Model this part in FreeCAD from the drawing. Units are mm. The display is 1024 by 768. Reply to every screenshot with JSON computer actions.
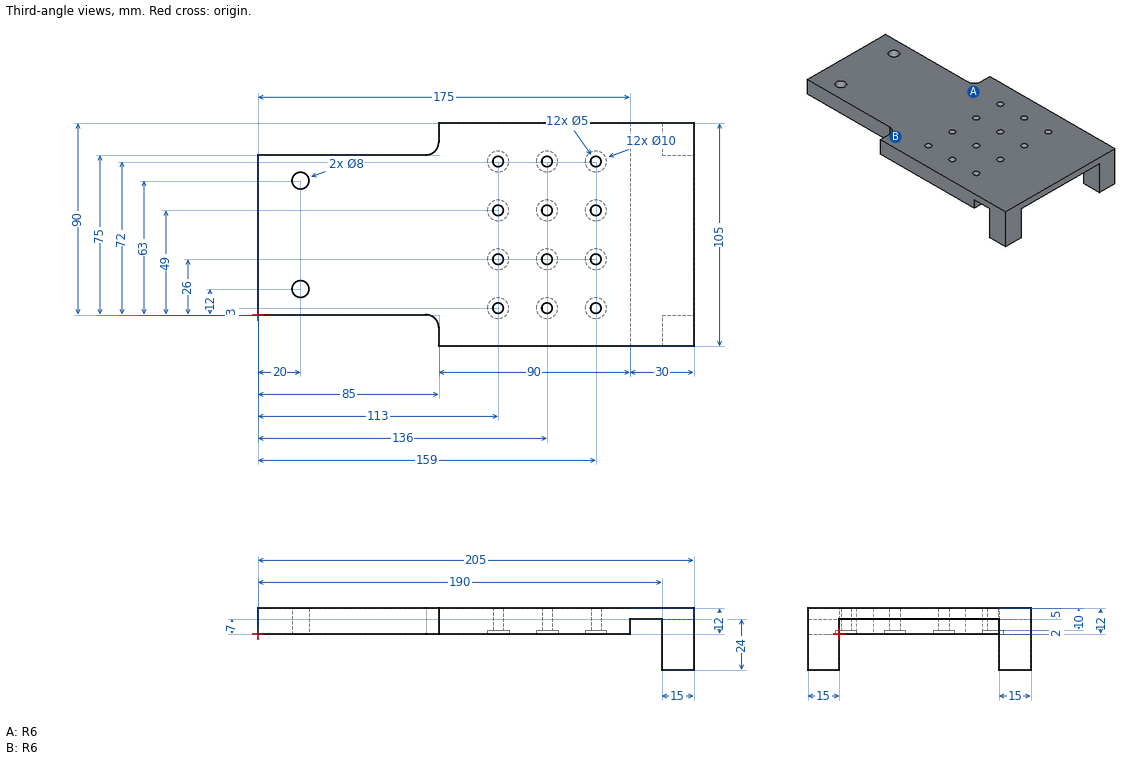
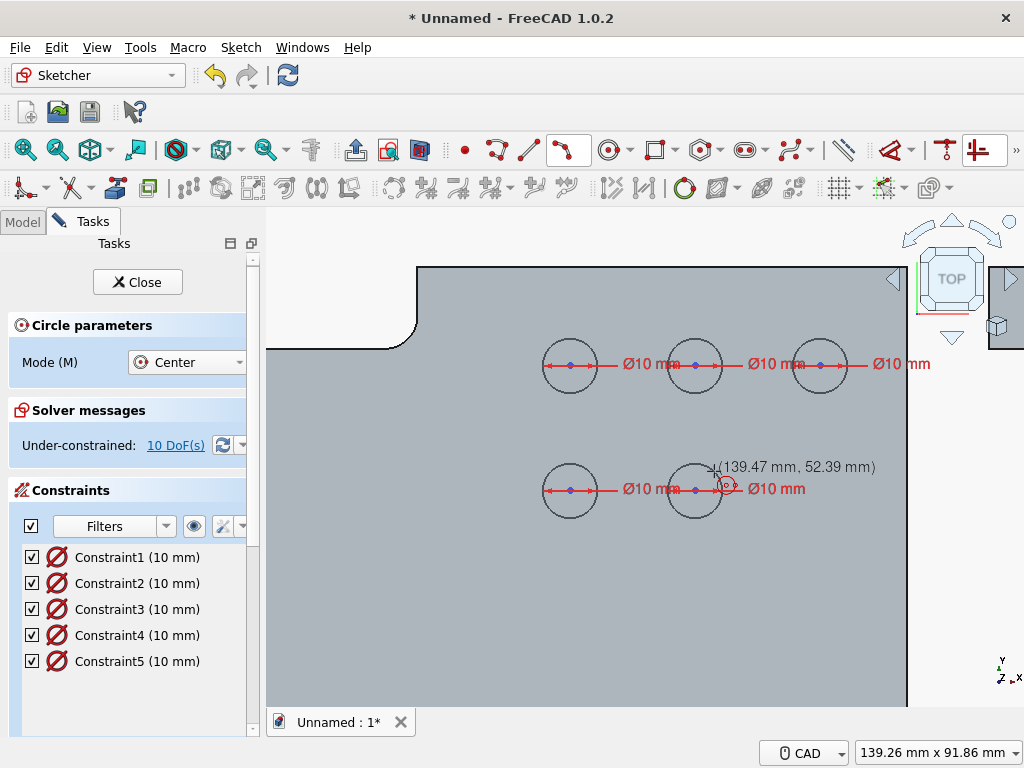
{"action": "left_click", "coordinate": [820, 490]}
{"action": "mouse_move", "coordinate": [840, 471]}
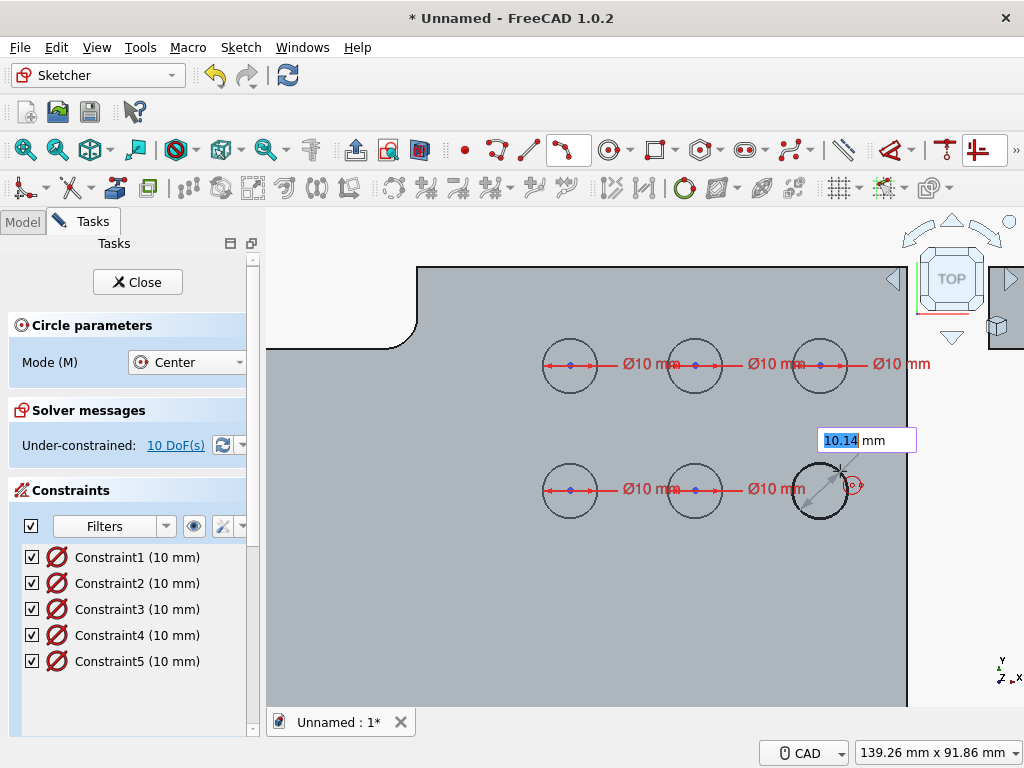
{"action": "type", "text": "10"}
{"action": "key", "text": "Return"}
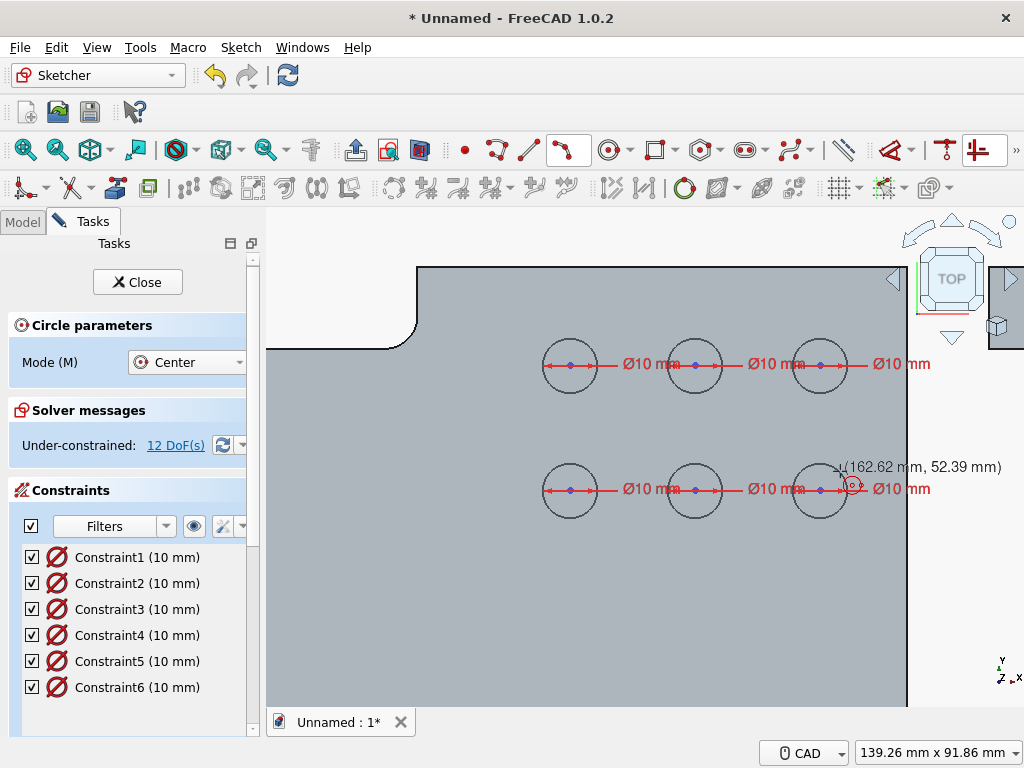
{"action": "left_click", "coordinate": [820, 616]}
{"action": "mouse_move", "coordinate": [840, 596]}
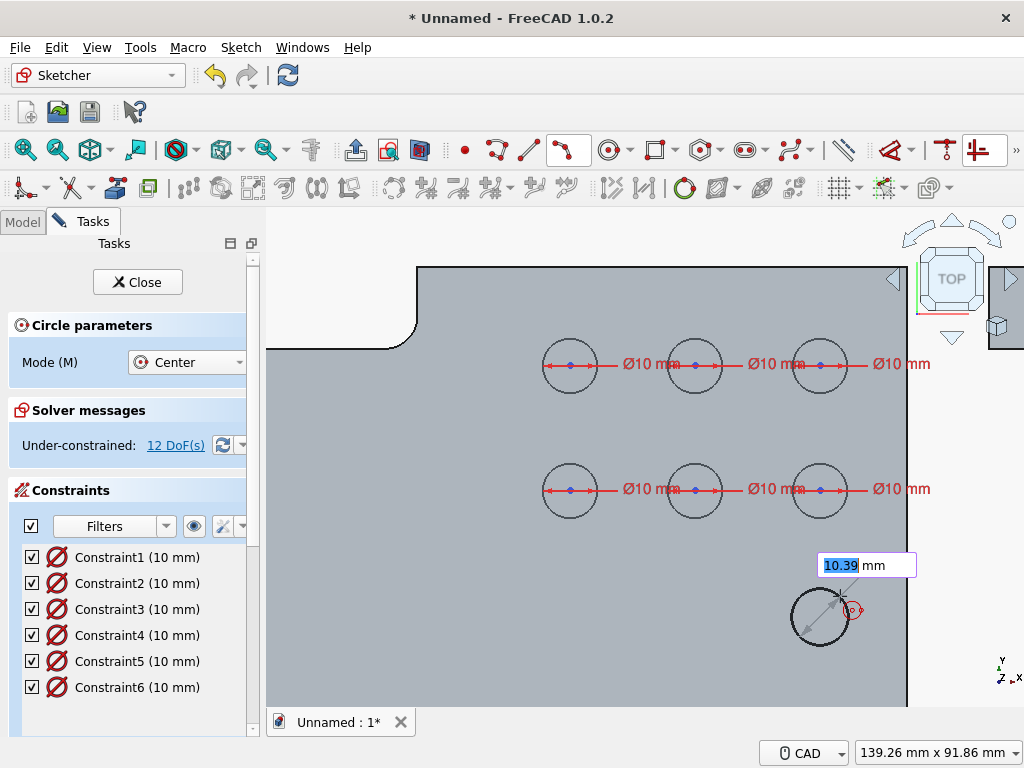
{"action": "type", "text": "10"}
{"action": "key", "text": "Return"}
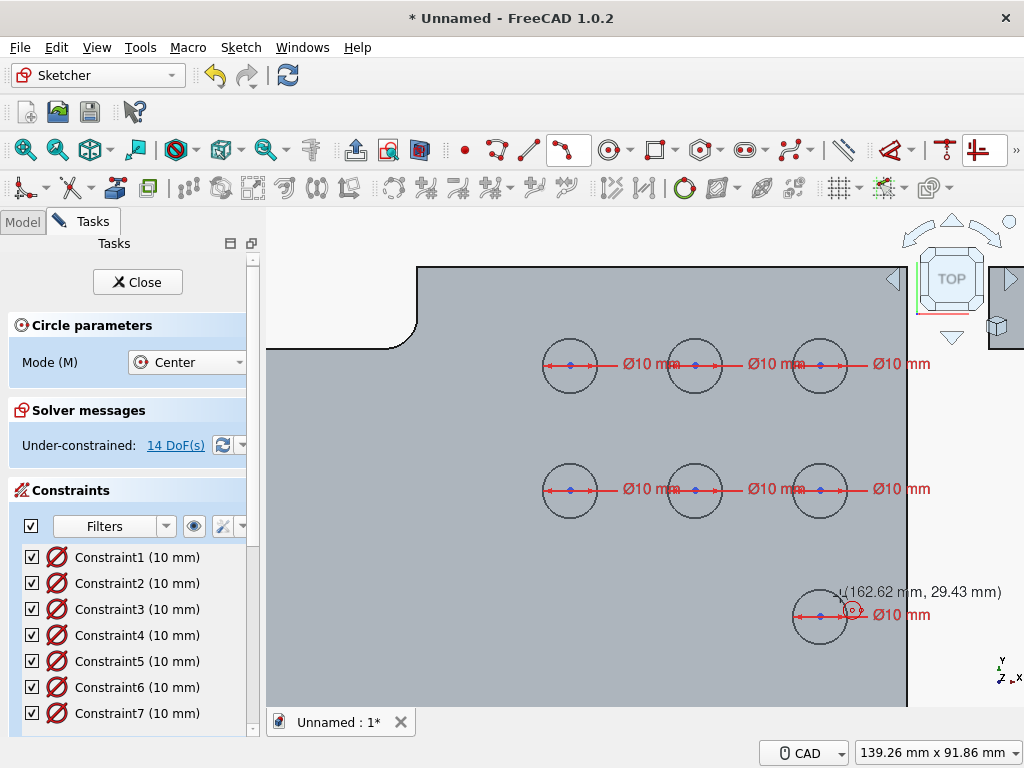
{"action": "left_click", "coordinate": [695, 616]}
{"action": "mouse_move", "coordinate": [714, 596]}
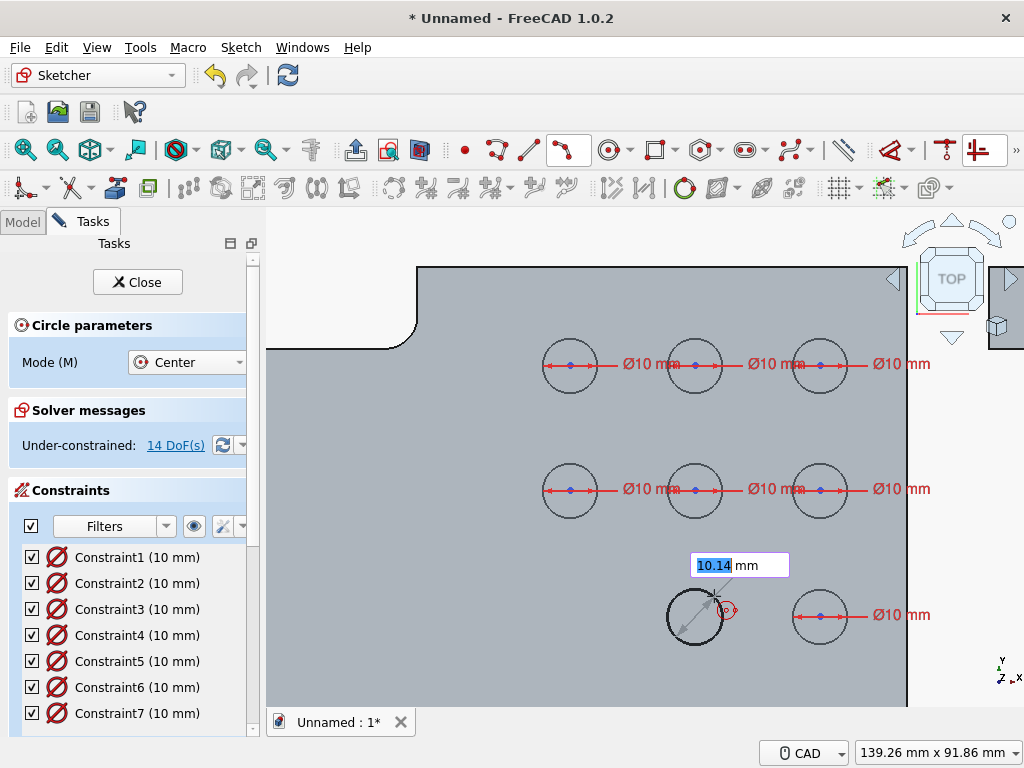
{"action": "type", "text": "10"}
{"action": "key", "text": "Return"}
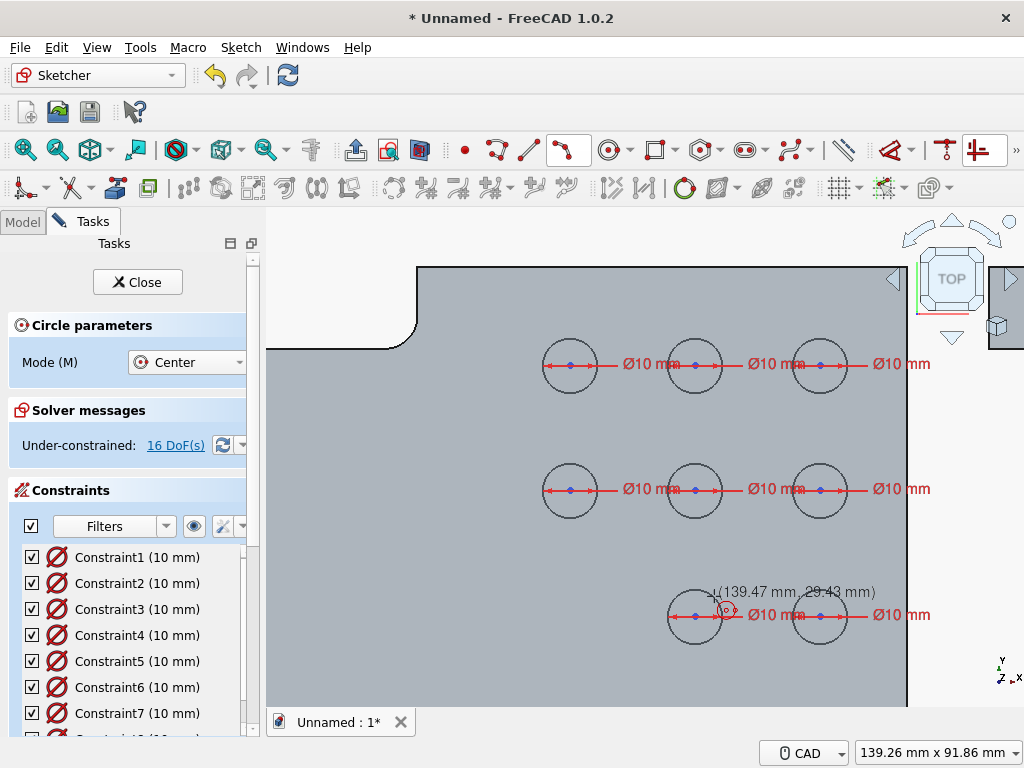
{"action": "left_click", "coordinate": [570, 616]}
{"action": "mouse_move", "coordinate": [589, 596]}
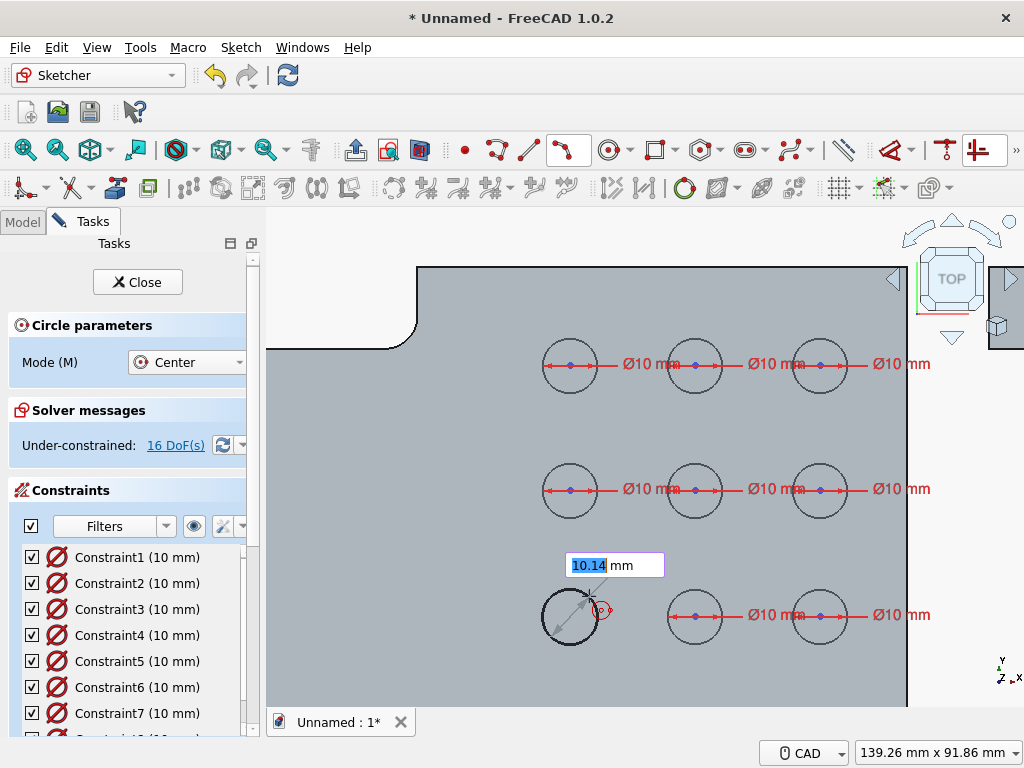
{"action": "type", "text": "10"}
{"action": "key", "text": "Return"}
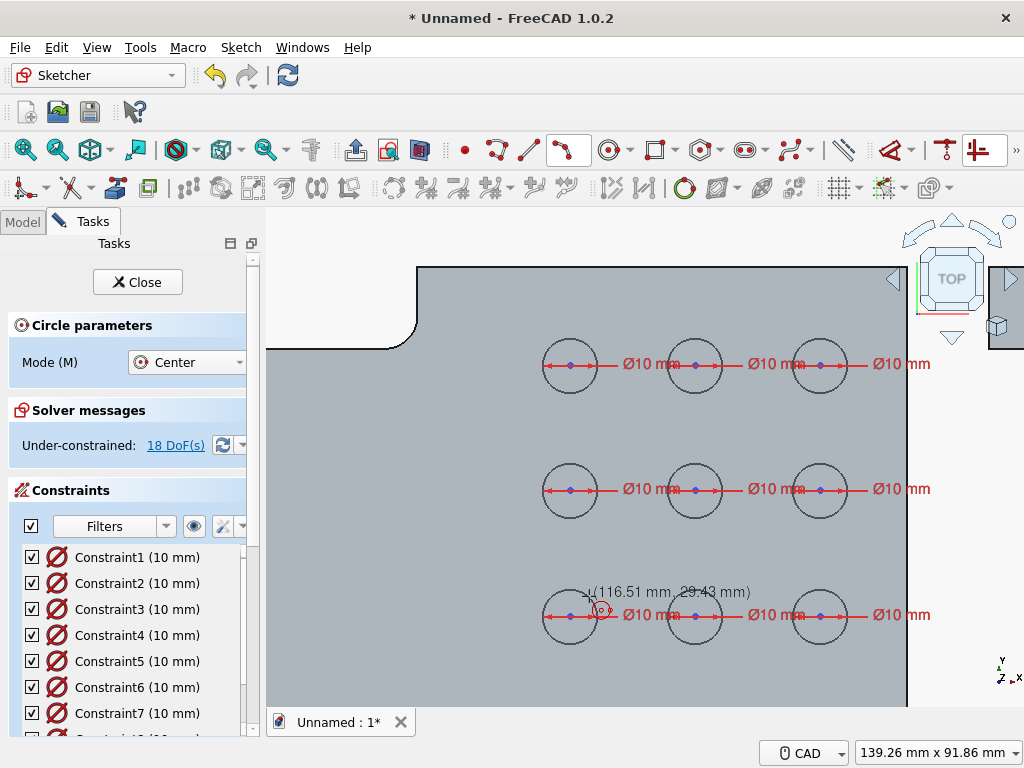
{"action": "scroll", "coordinate": [720, 379], "scroll_direction": "down", "scroll_amount": 4}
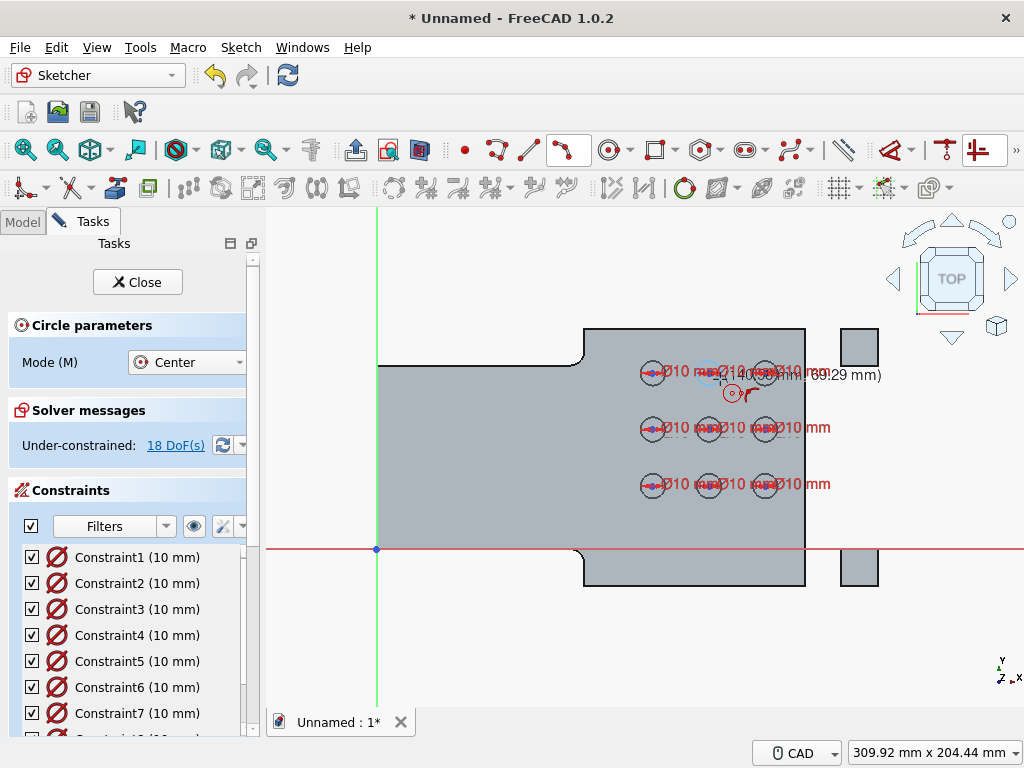
{"action": "scroll", "coordinate": [653, 542], "scroll_direction": "up", "scroll_amount": 4}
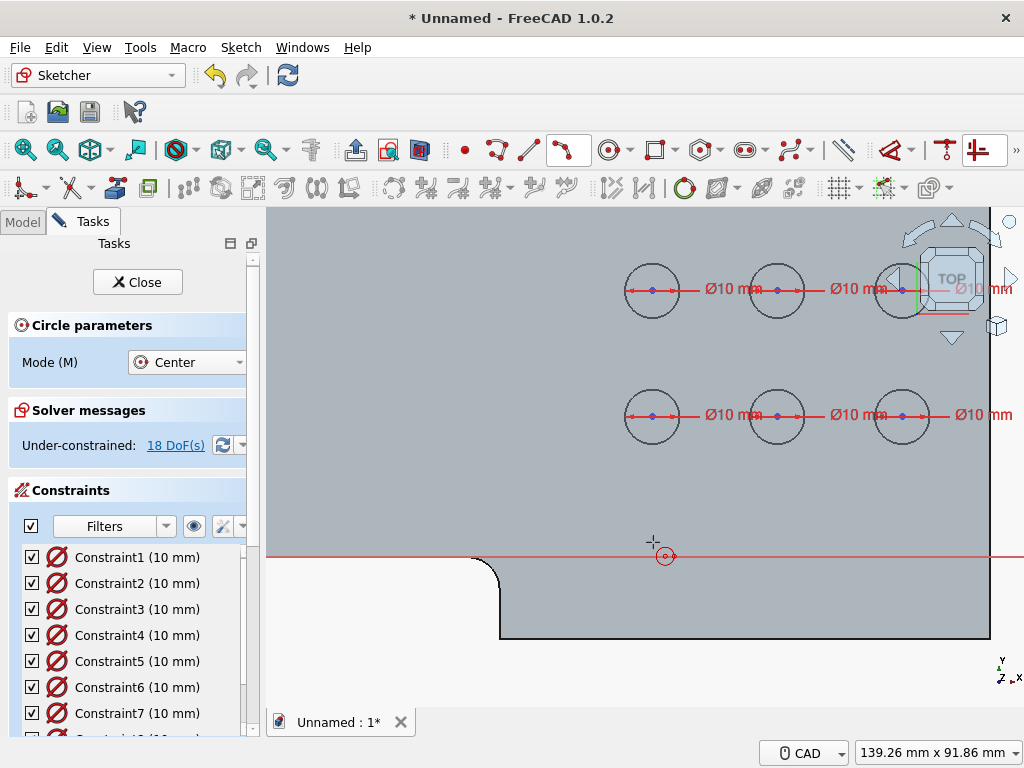
{"action": "left_click", "coordinate": [652, 541]}
{"action": "mouse_move", "coordinate": [671, 521]}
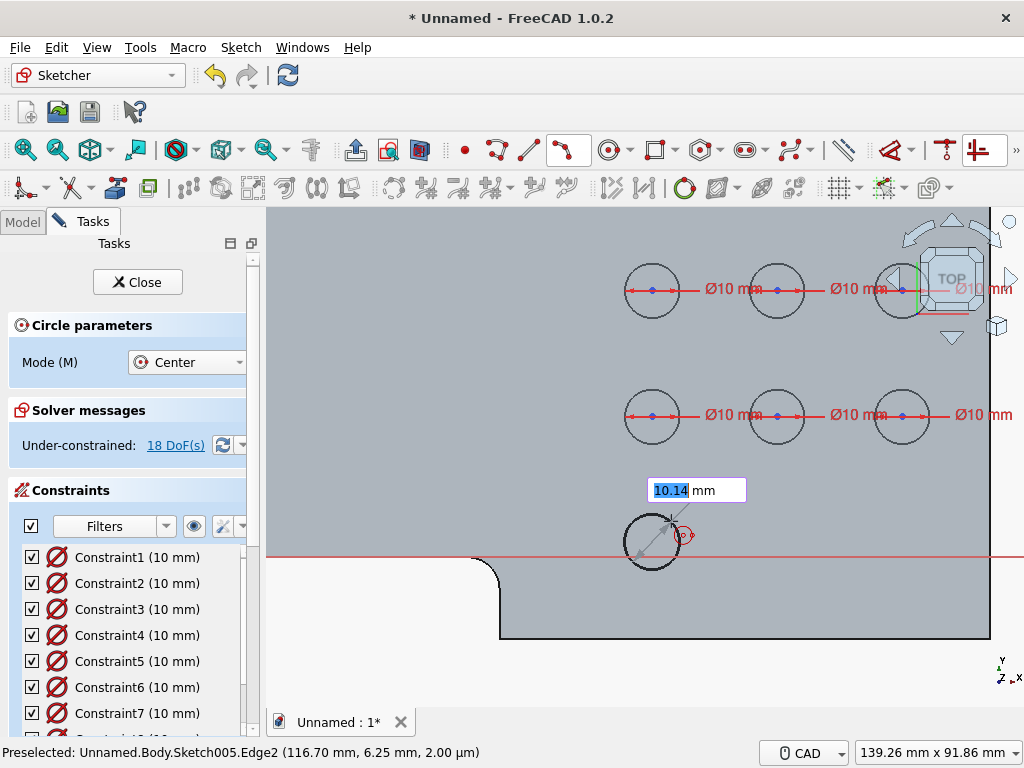
{"action": "type", "text": "10"}
{"action": "key", "text": "Return"}